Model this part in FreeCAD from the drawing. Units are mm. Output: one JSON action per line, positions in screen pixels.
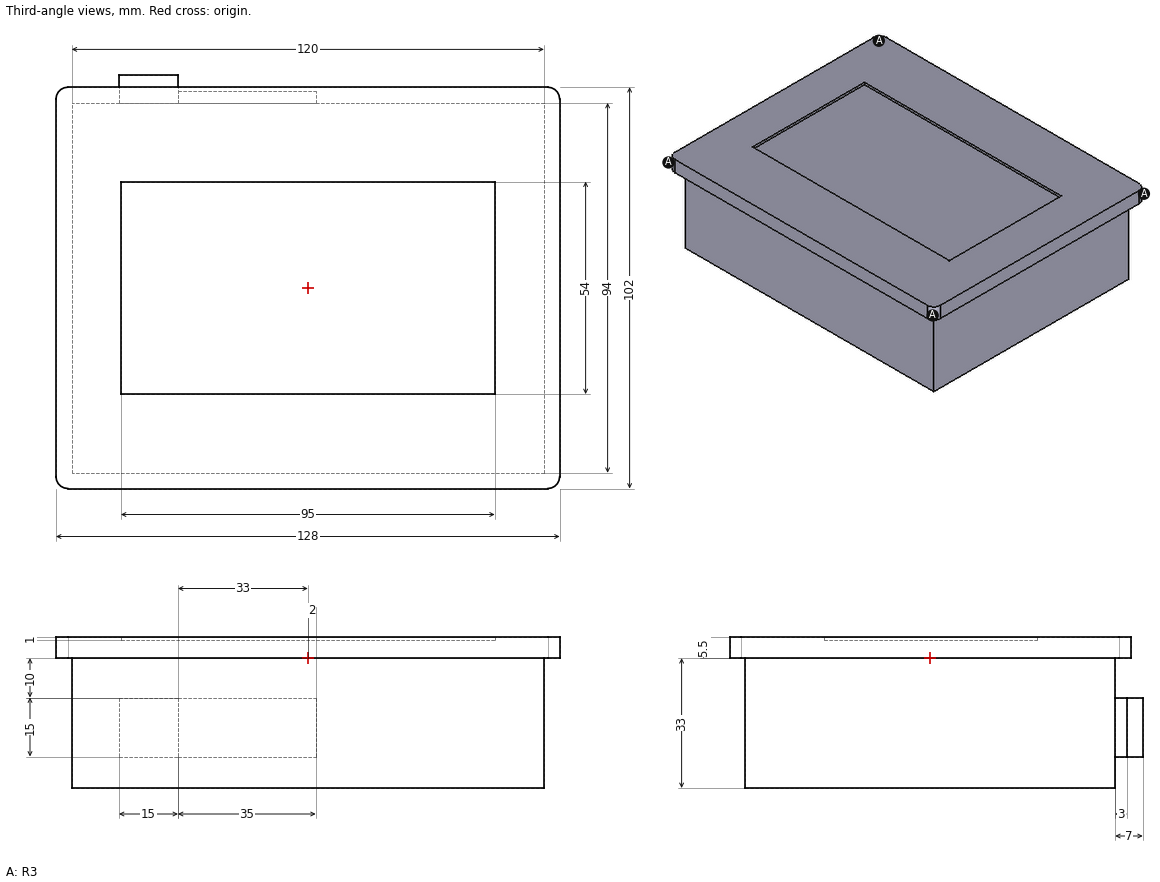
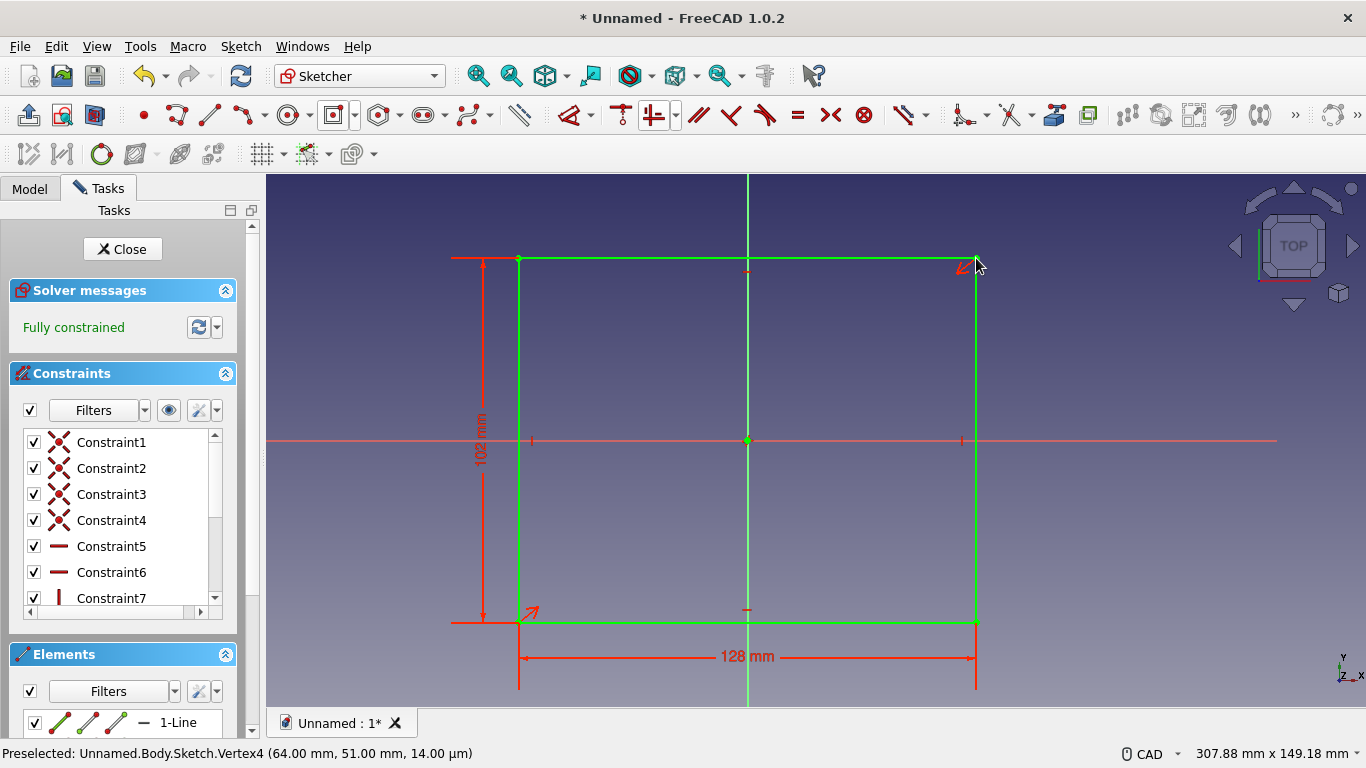
{"action": "left_click", "coordinate": [123, 249]}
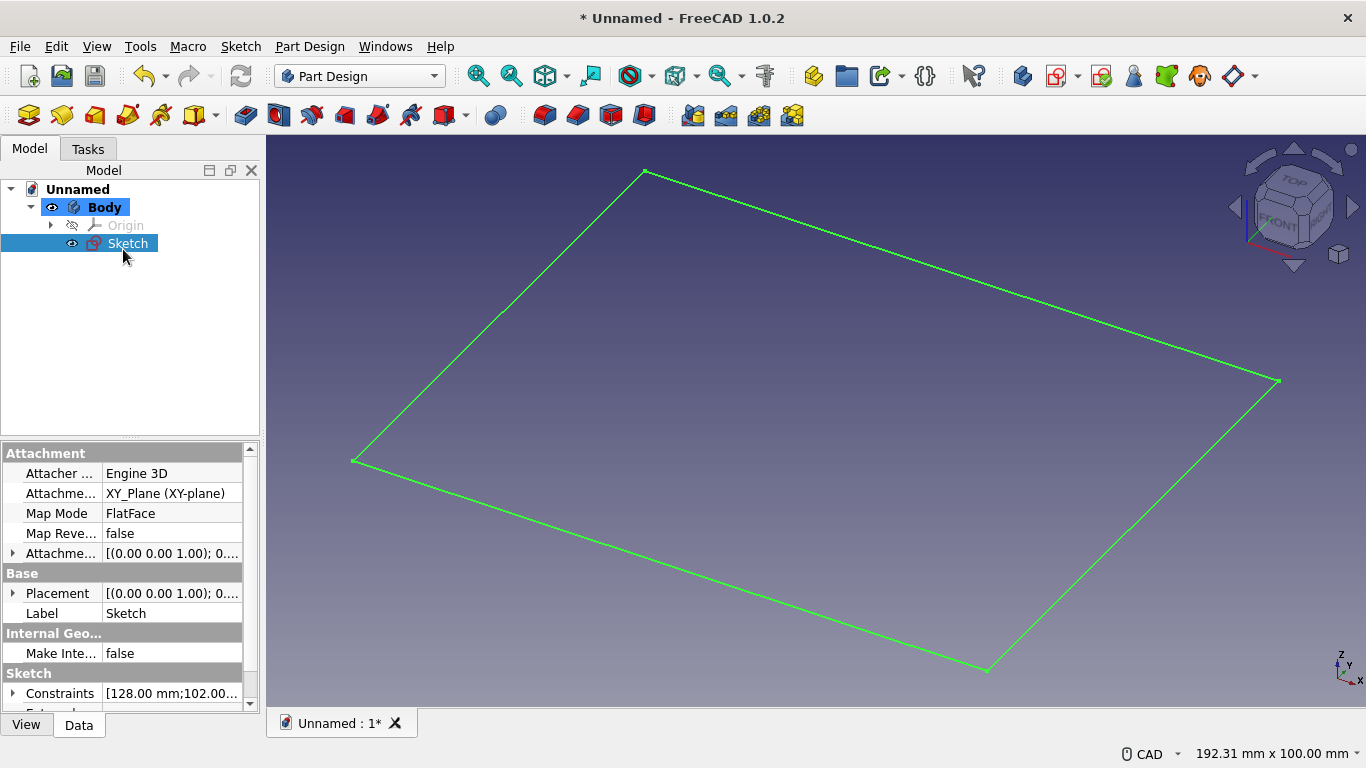
{"action": "left_click", "coordinate": [29, 116]}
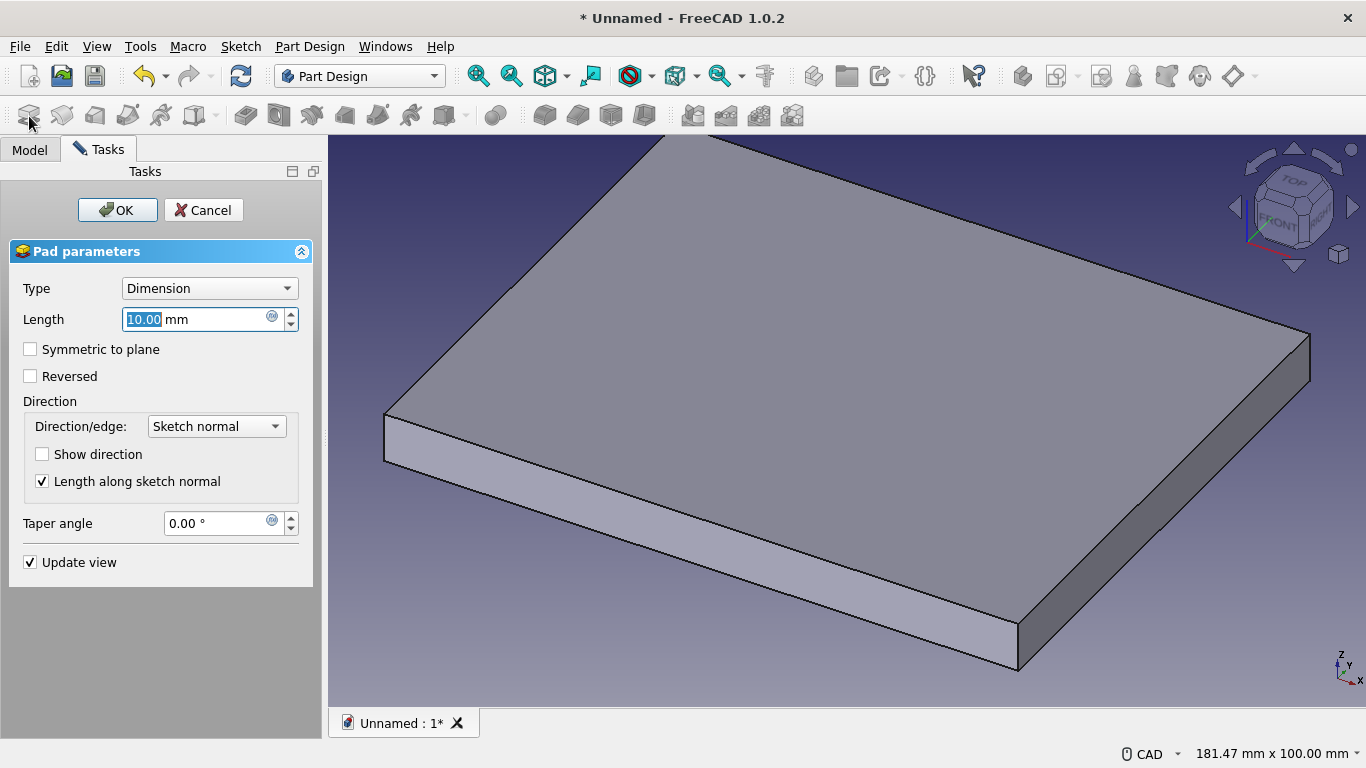
{"action": "type", "text": "5.5"}
{"action": "key", "text": "Tab"}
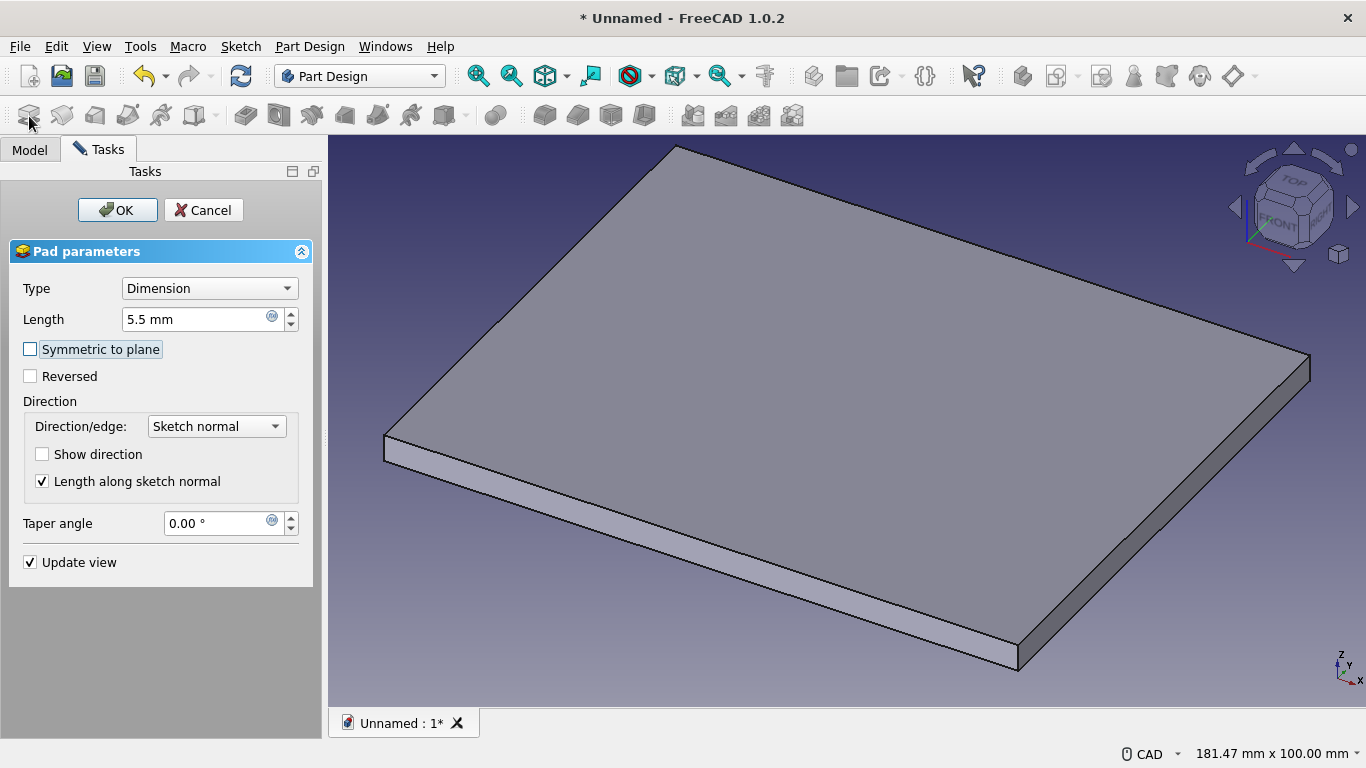
{"action": "left_click", "coordinate": [118, 210]}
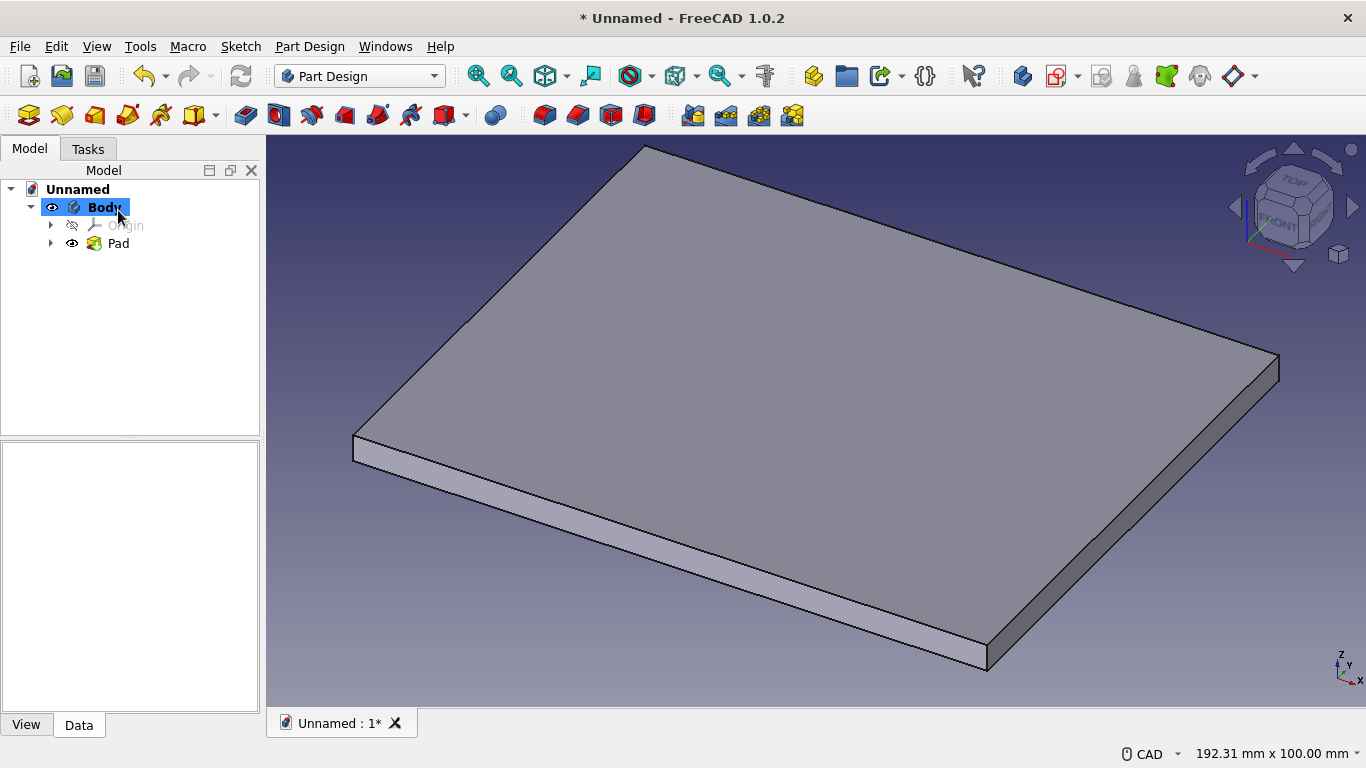
{"action": "left_click", "coordinate": [816, 394]}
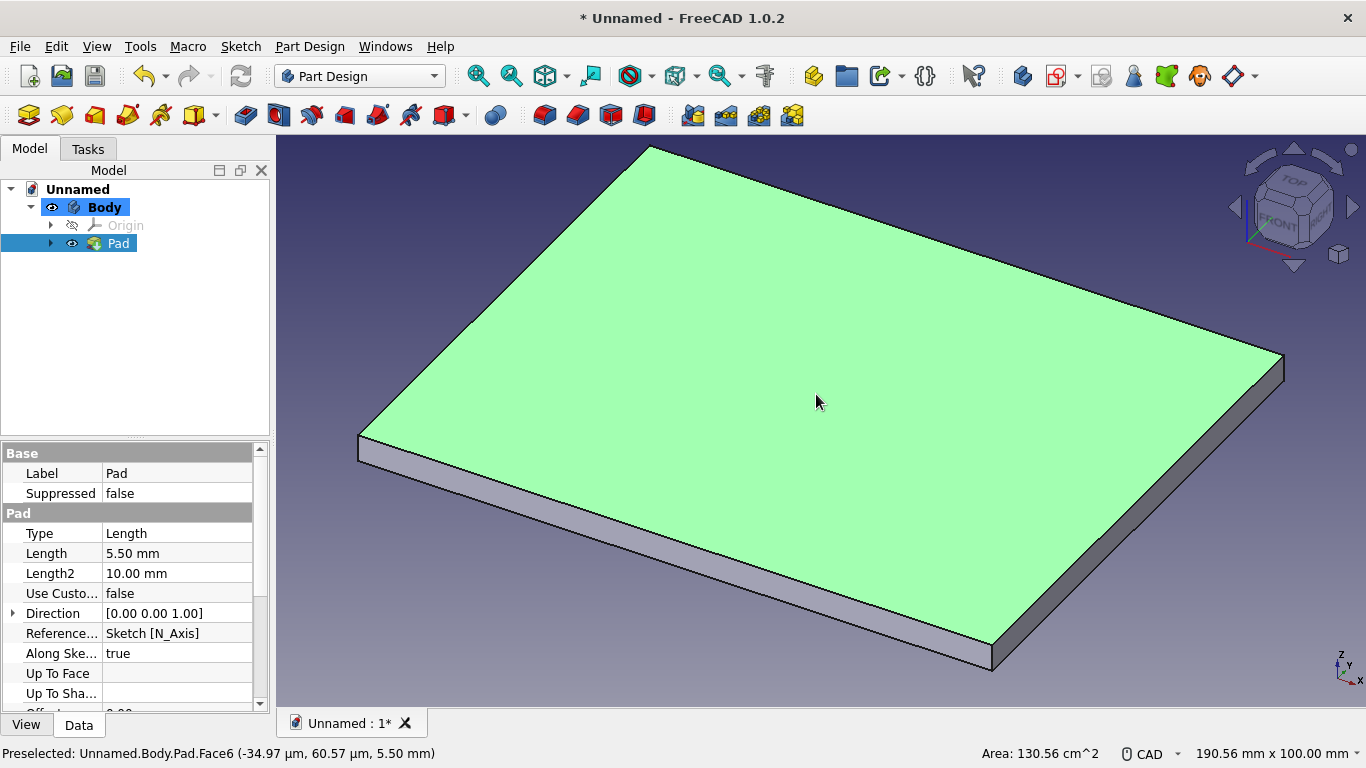
{"action": "left_click", "coordinate": [1056, 76]}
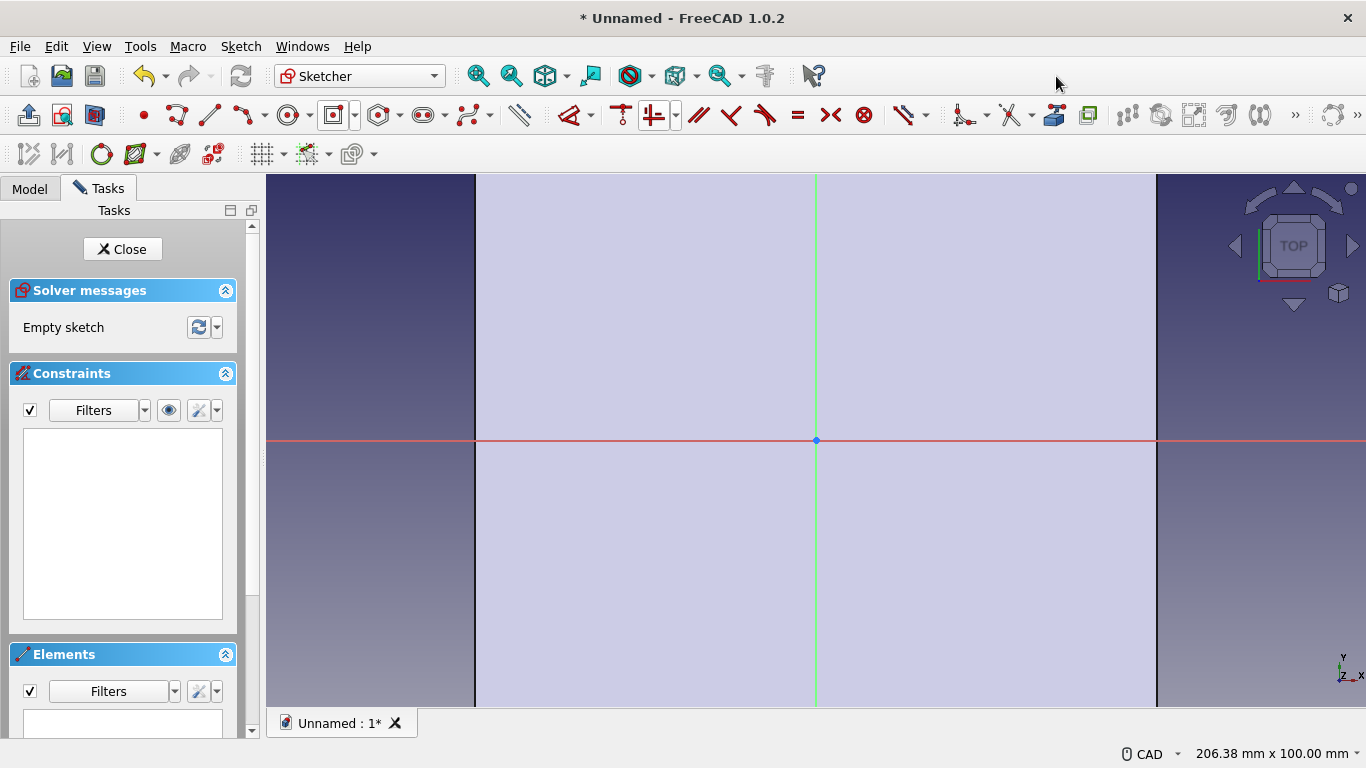
{"action": "left_click", "coordinate": [332, 116]}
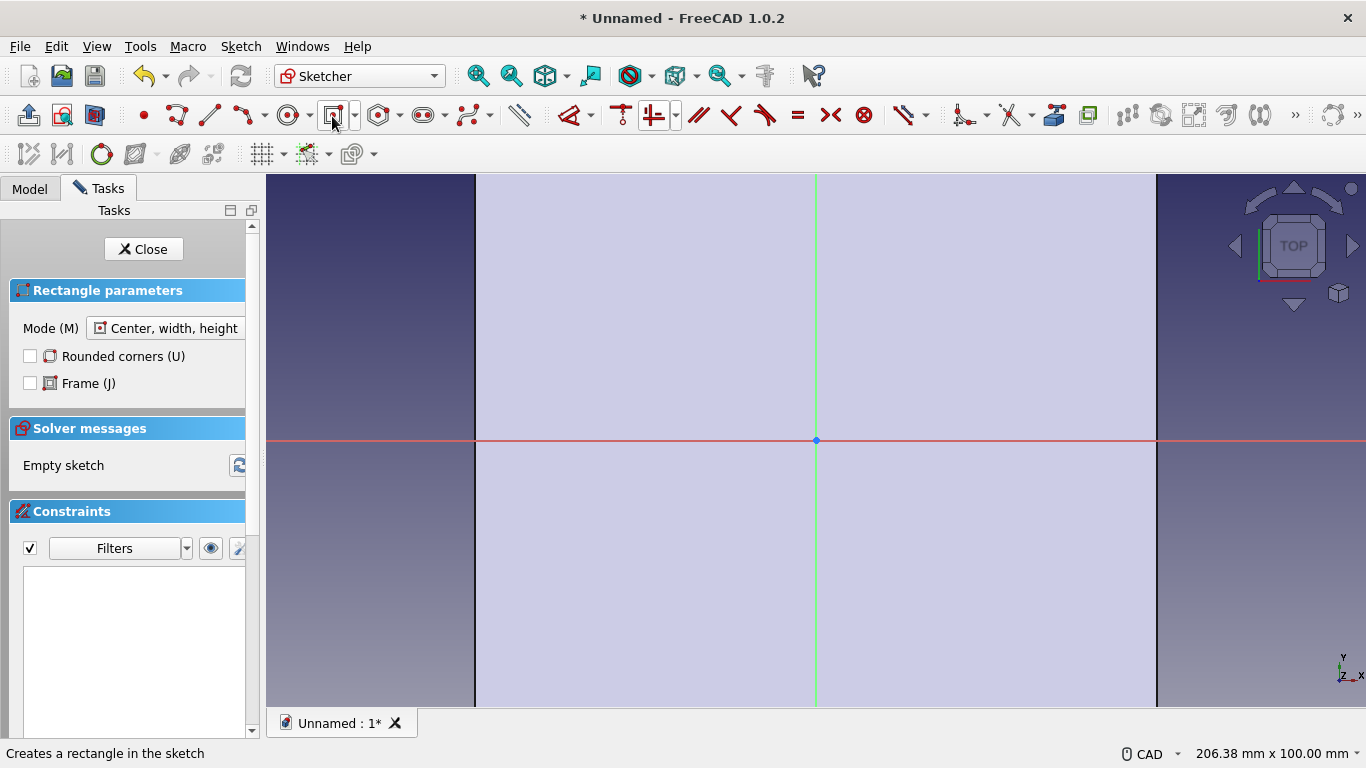
{"action": "left_click", "coordinate": [816, 440]}
{"action": "mouse_move", "coordinate": [1069, 297]}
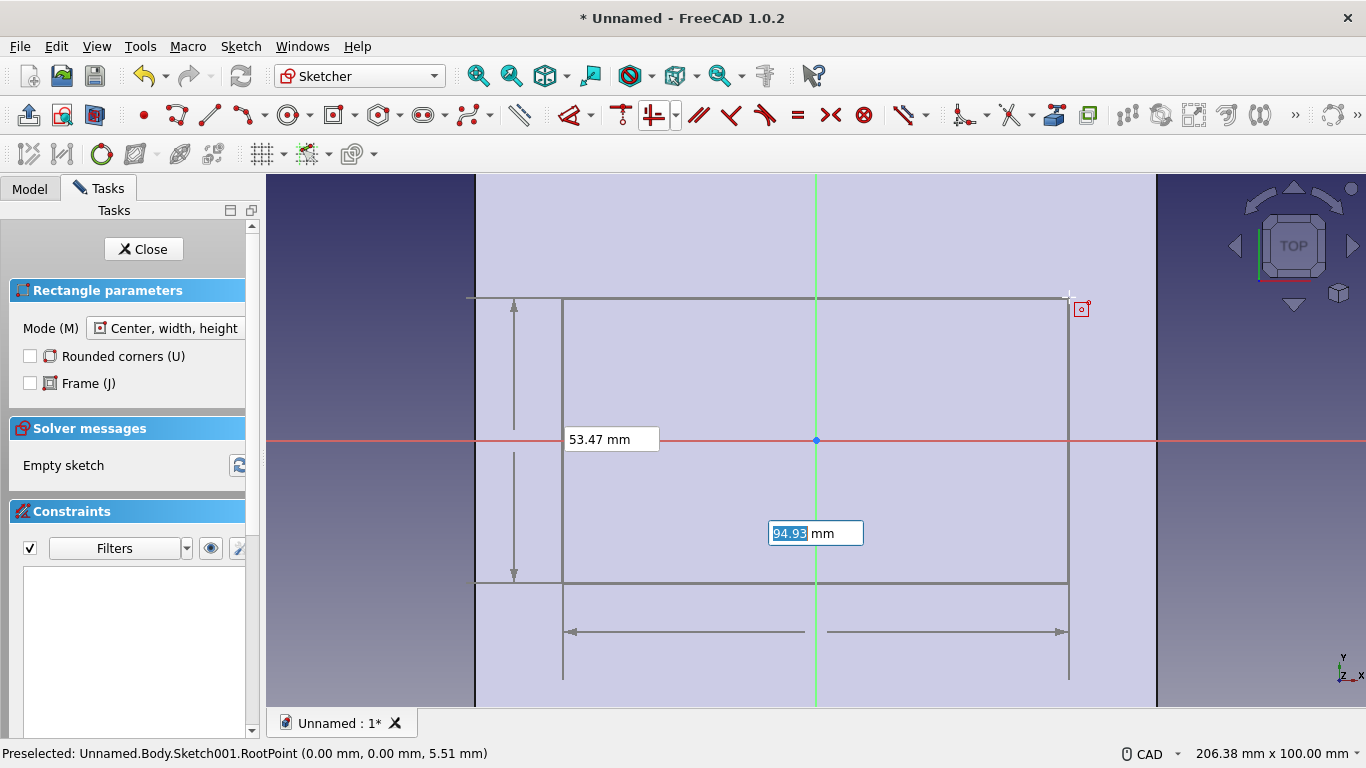
{"action": "type", "text": "95"}
{"action": "key", "text": "Tab"}
{"action": "type", "text": "54"}
{"action": "key", "text": "Return"}
{"action": "key", "text": "Escape"}